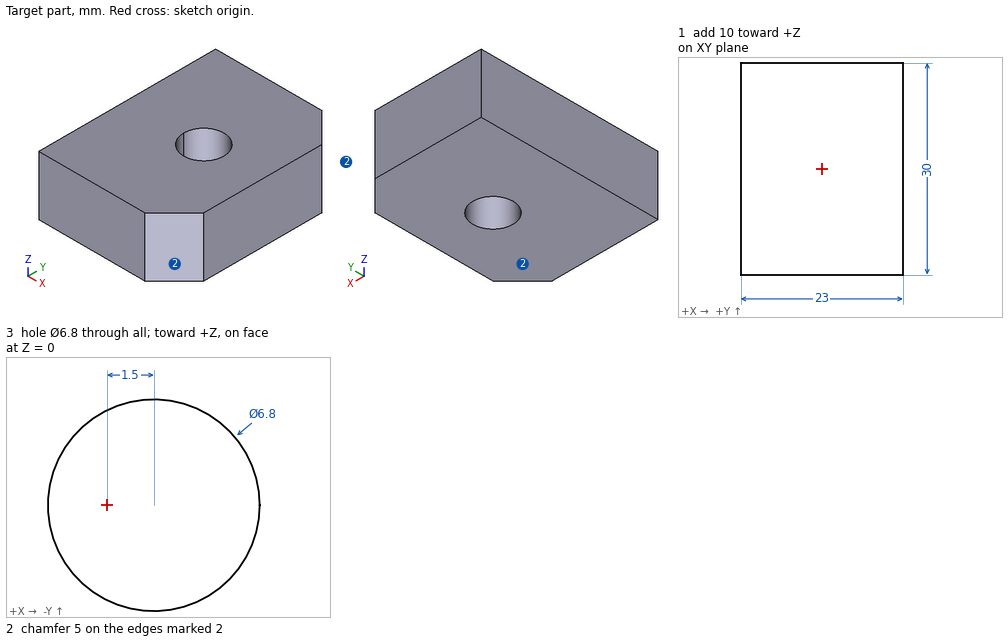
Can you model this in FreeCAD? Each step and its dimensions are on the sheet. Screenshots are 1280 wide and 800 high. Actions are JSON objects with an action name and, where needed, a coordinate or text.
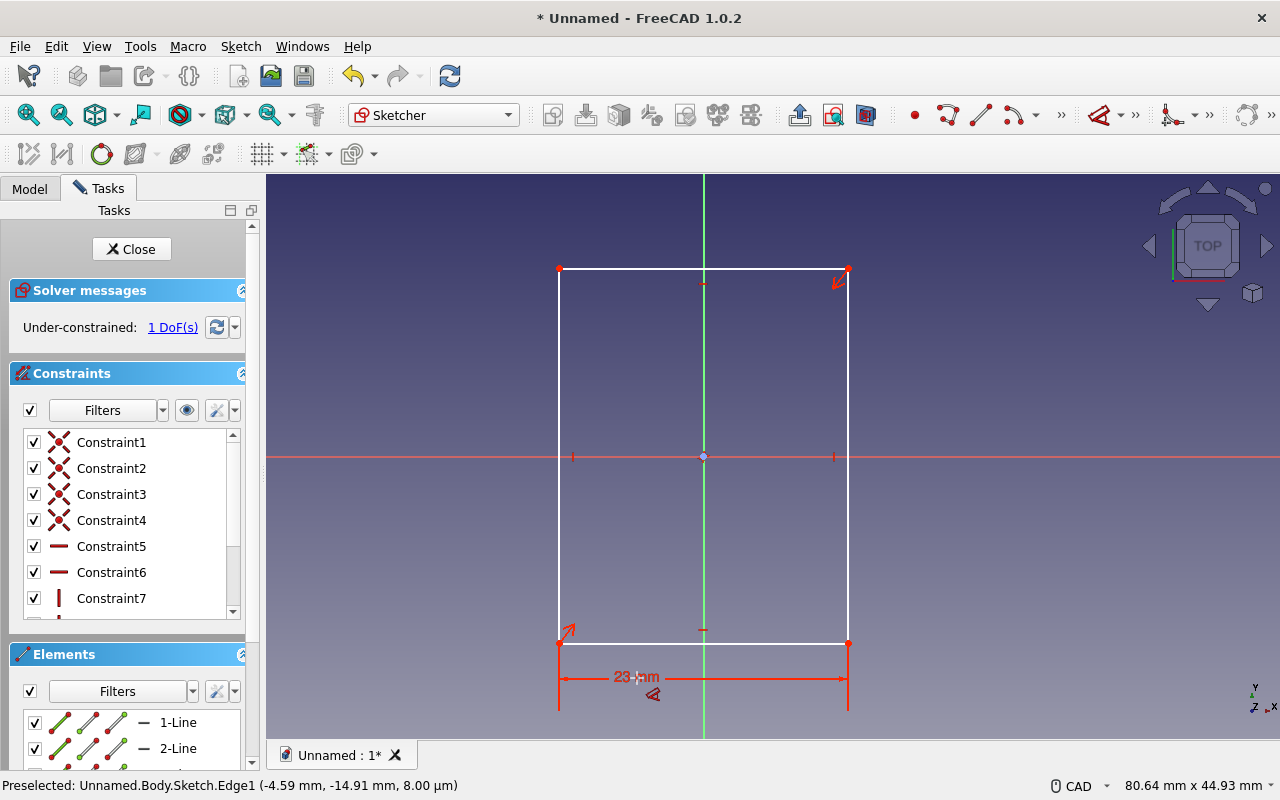
{"action": "left_click", "coordinate": [848, 531]}
{"action": "left_click", "coordinate": [882, 370]}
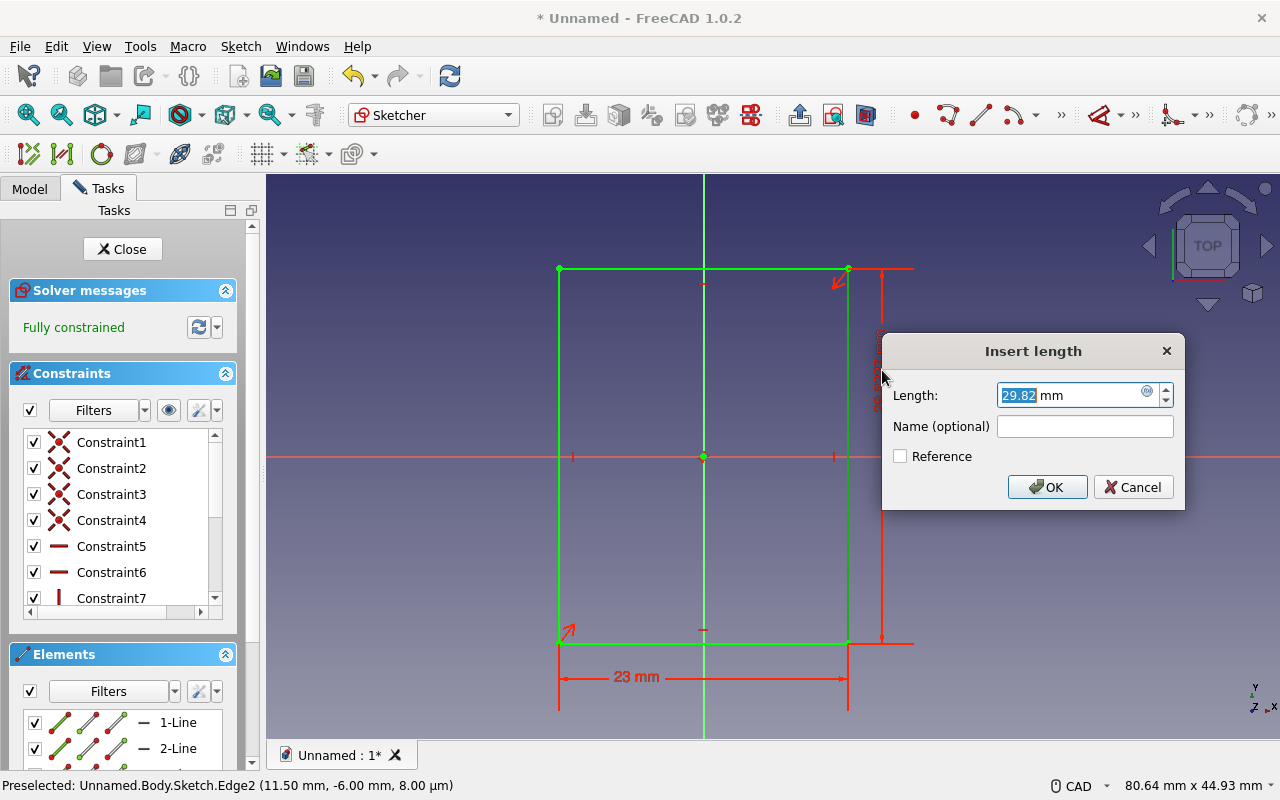
{"action": "type", "text": "30"}
{"action": "key", "text": "Return"}
{"action": "key", "text": "Escape"}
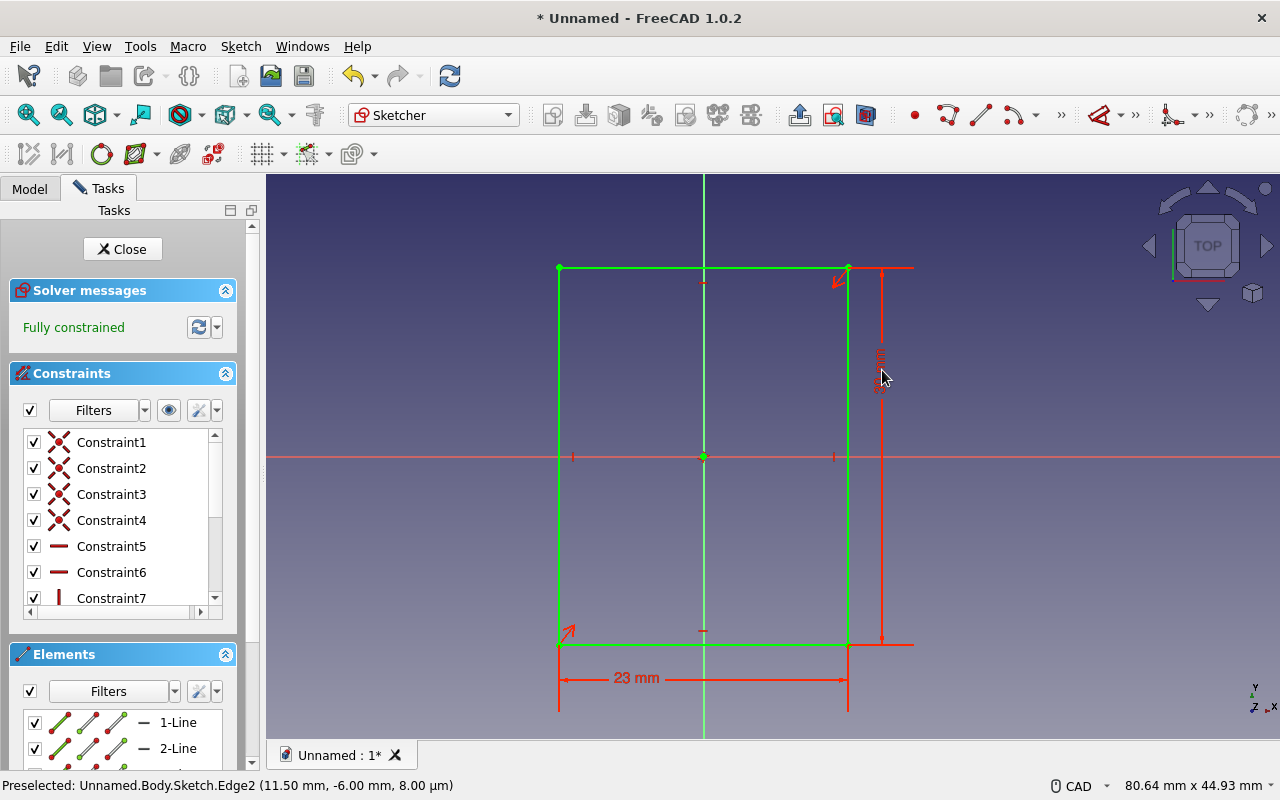
{"action": "left_click", "coordinate": [123, 249]}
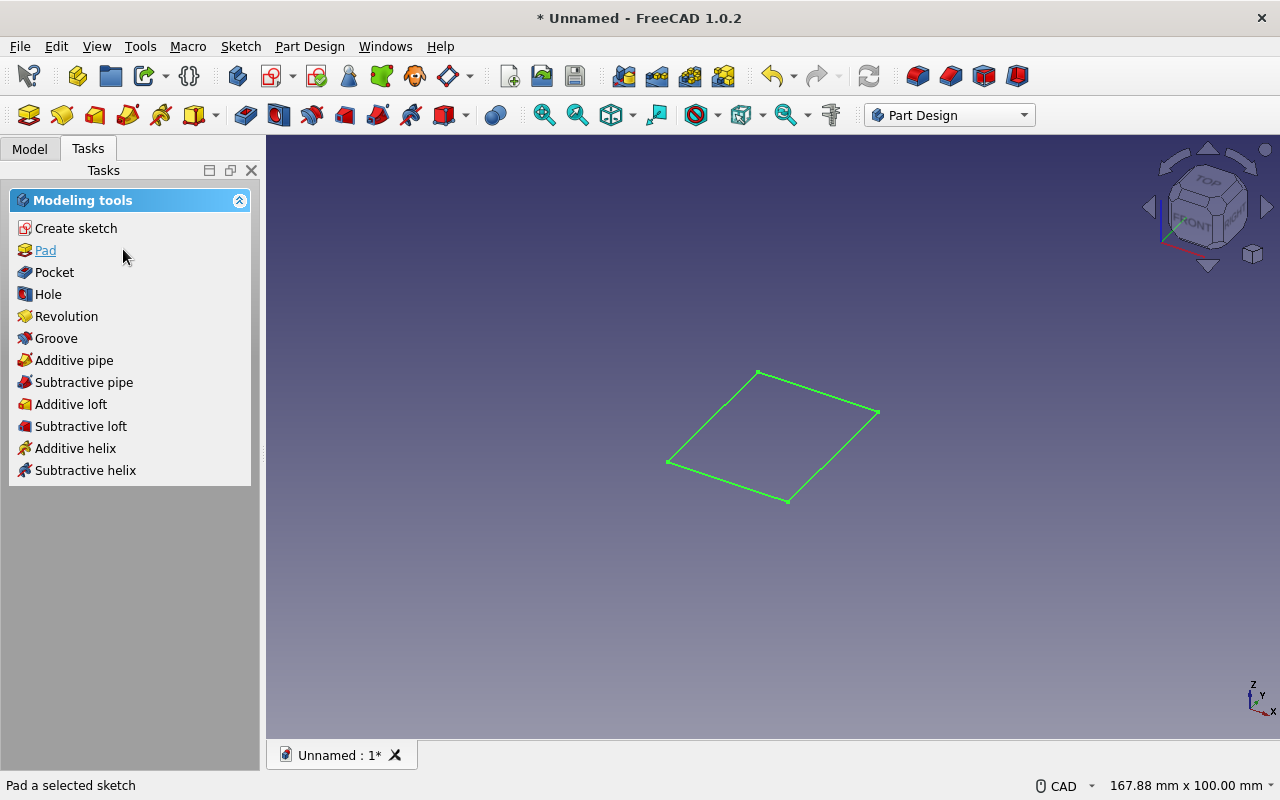
{"action": "left_click", "coordinate": [29, 116]}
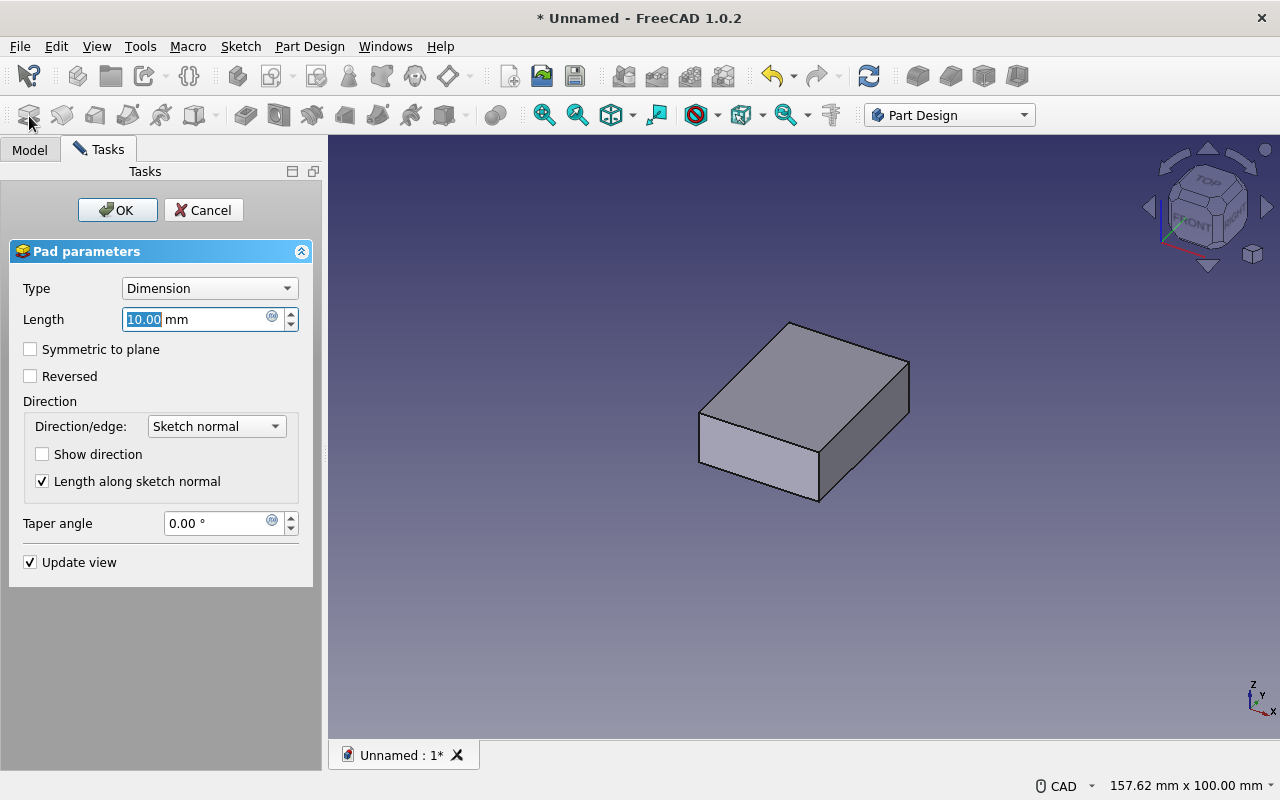
{"action": "type", "text": "10"}
{"action": "key", "text": "Tab"}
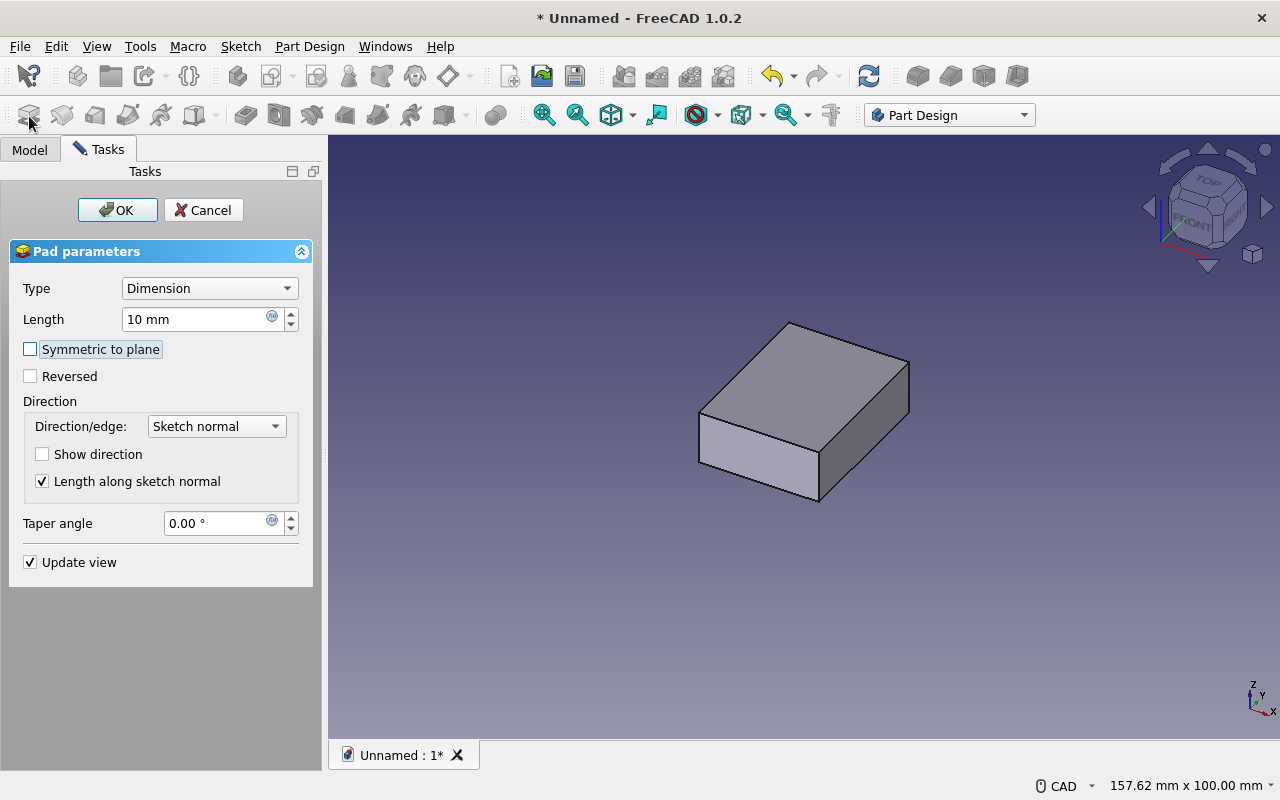
{"action": "left_click", "coordinate": [118, 210]}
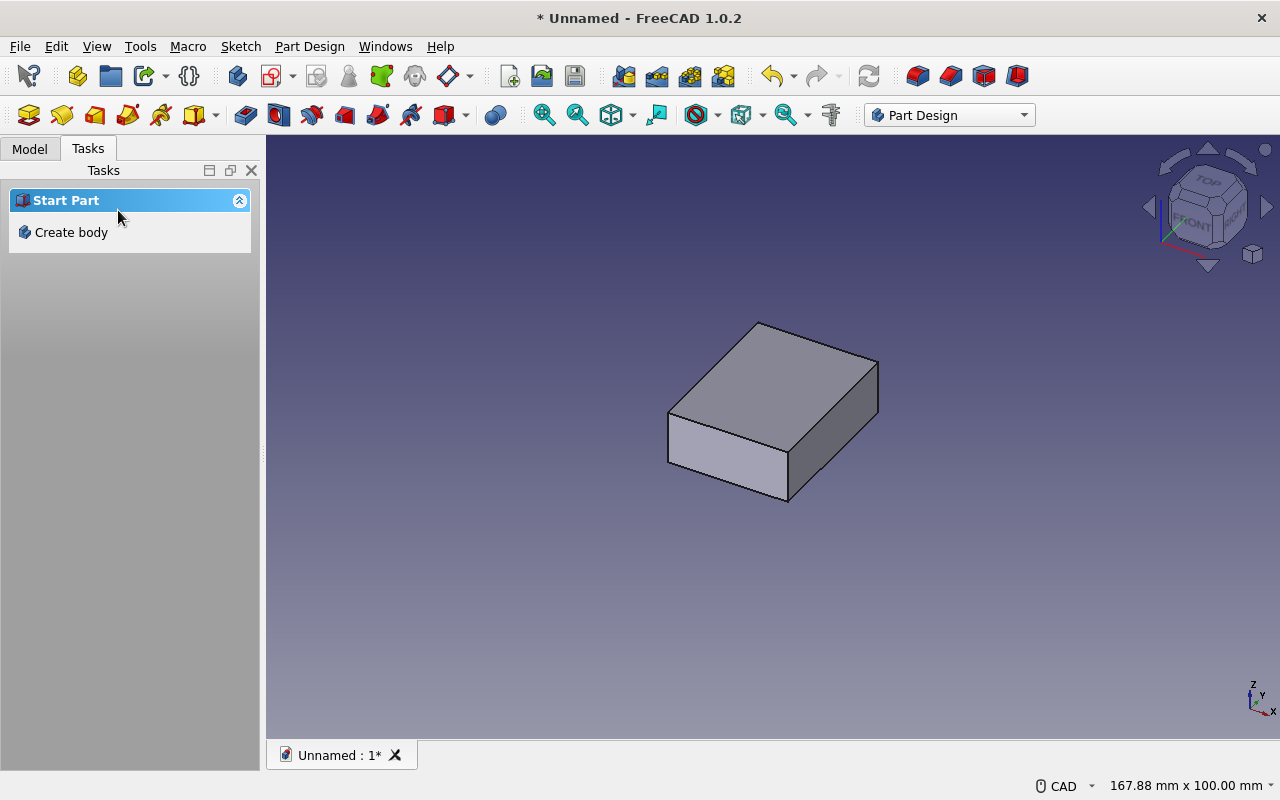
{"action": "left_click", "coordinate": [545, 116]}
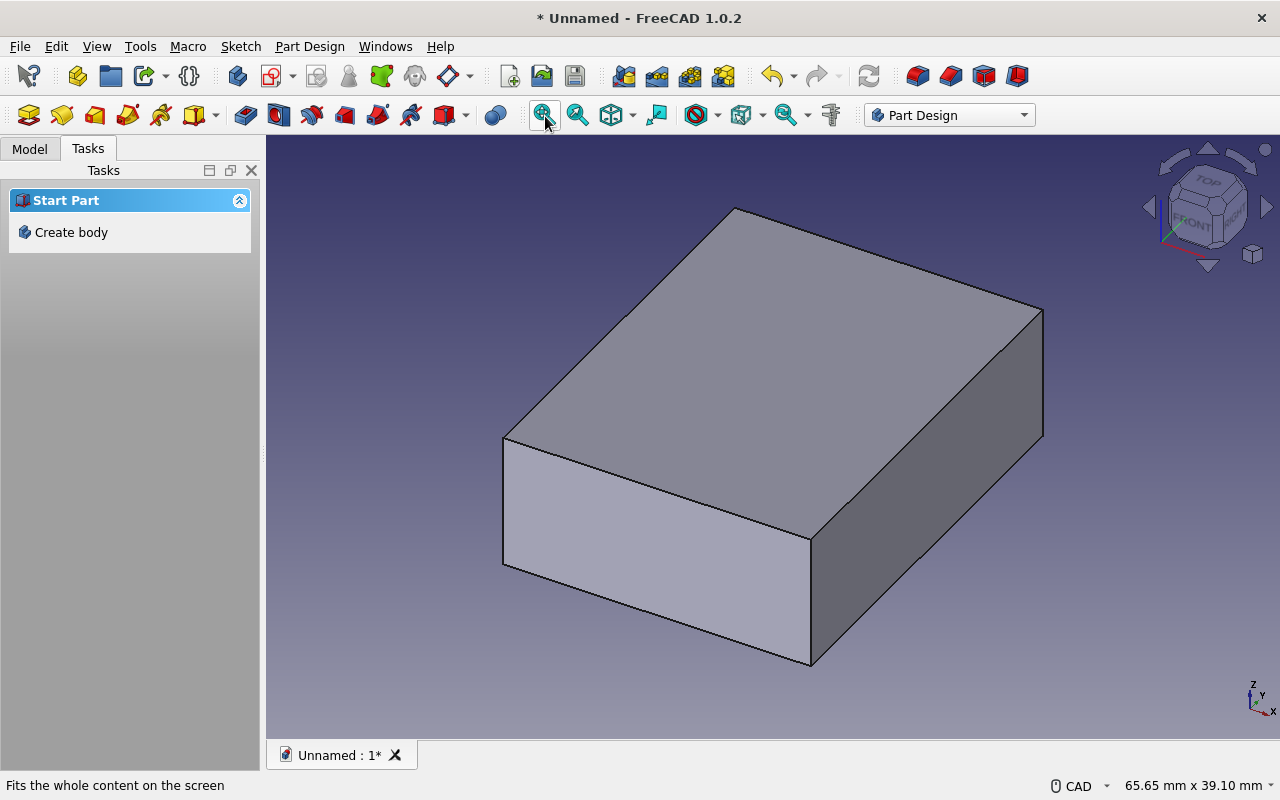
{"action": "left_click", "coordinate": [811, 602]}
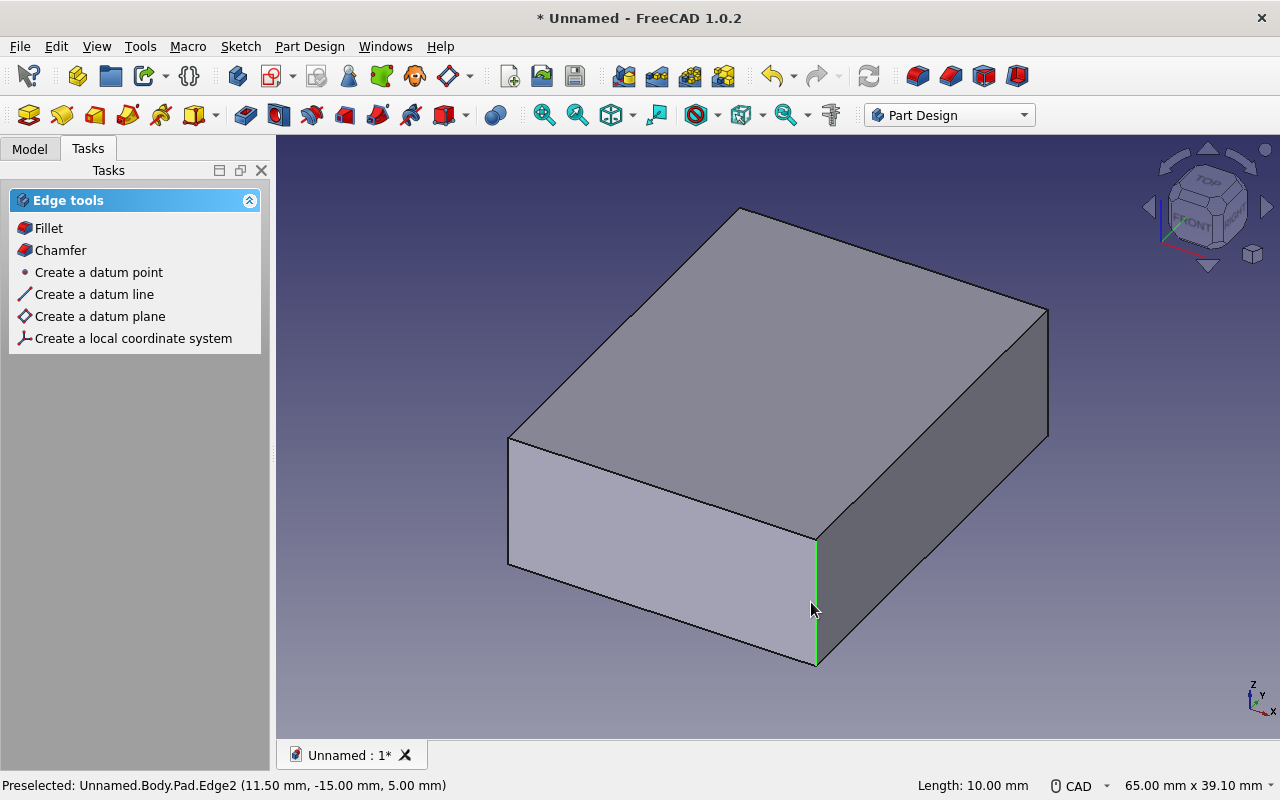
{"action": "key", "text": "0"}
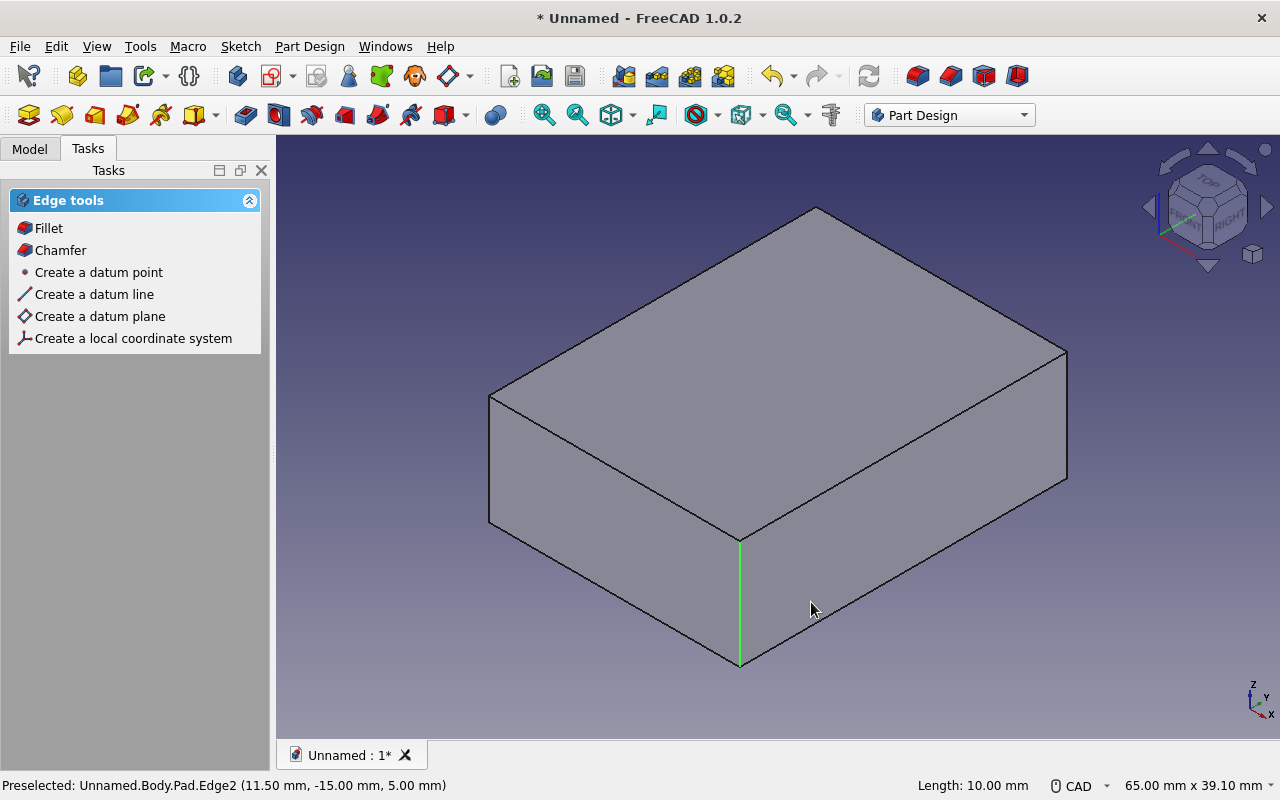
{"action": "key", "text": "2"}